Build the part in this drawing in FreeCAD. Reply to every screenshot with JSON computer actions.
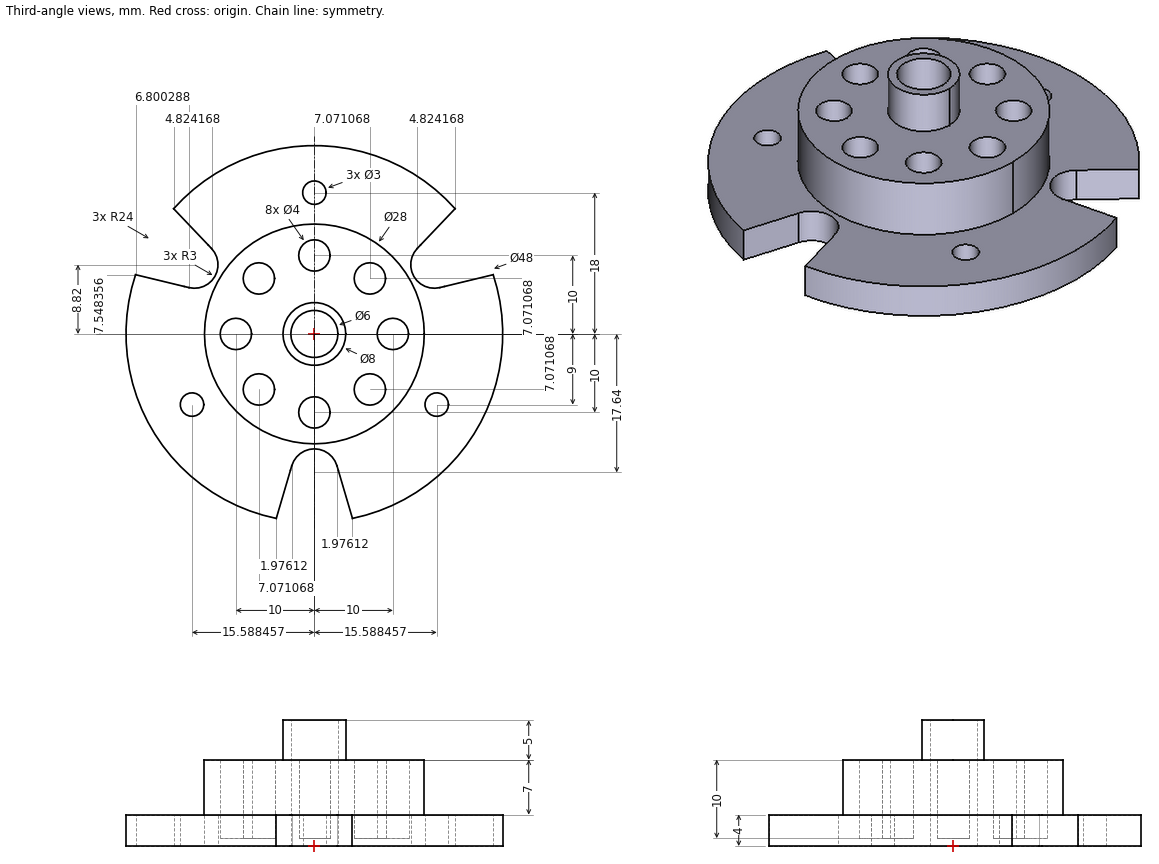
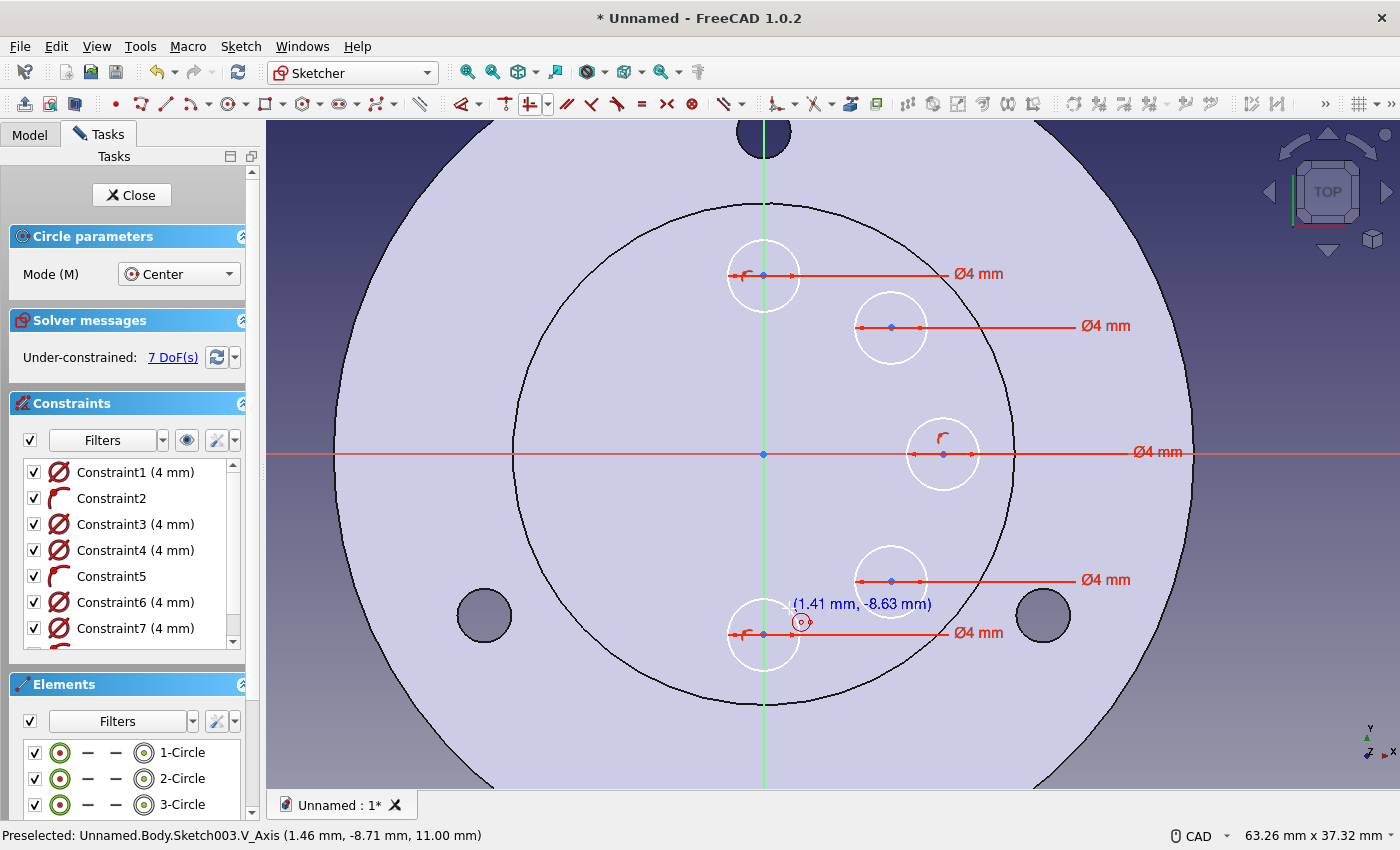
{"action": "left_click", "coordinate": [637, 581]}
{"action": "mouse_move", "coordinate": [662, 556]}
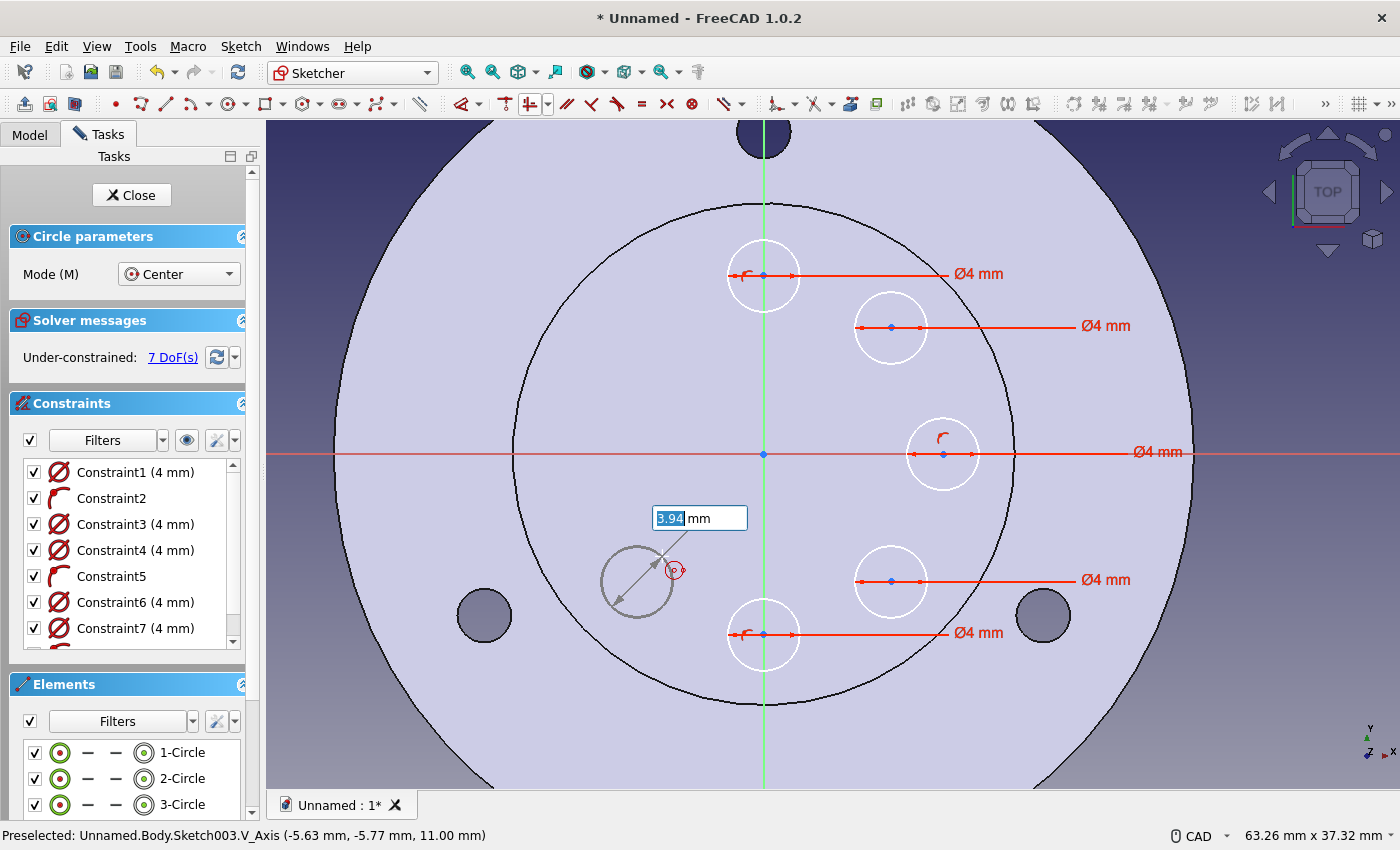
{"action": "type", "text": "4"}
{"action": "key", "text": "Return"}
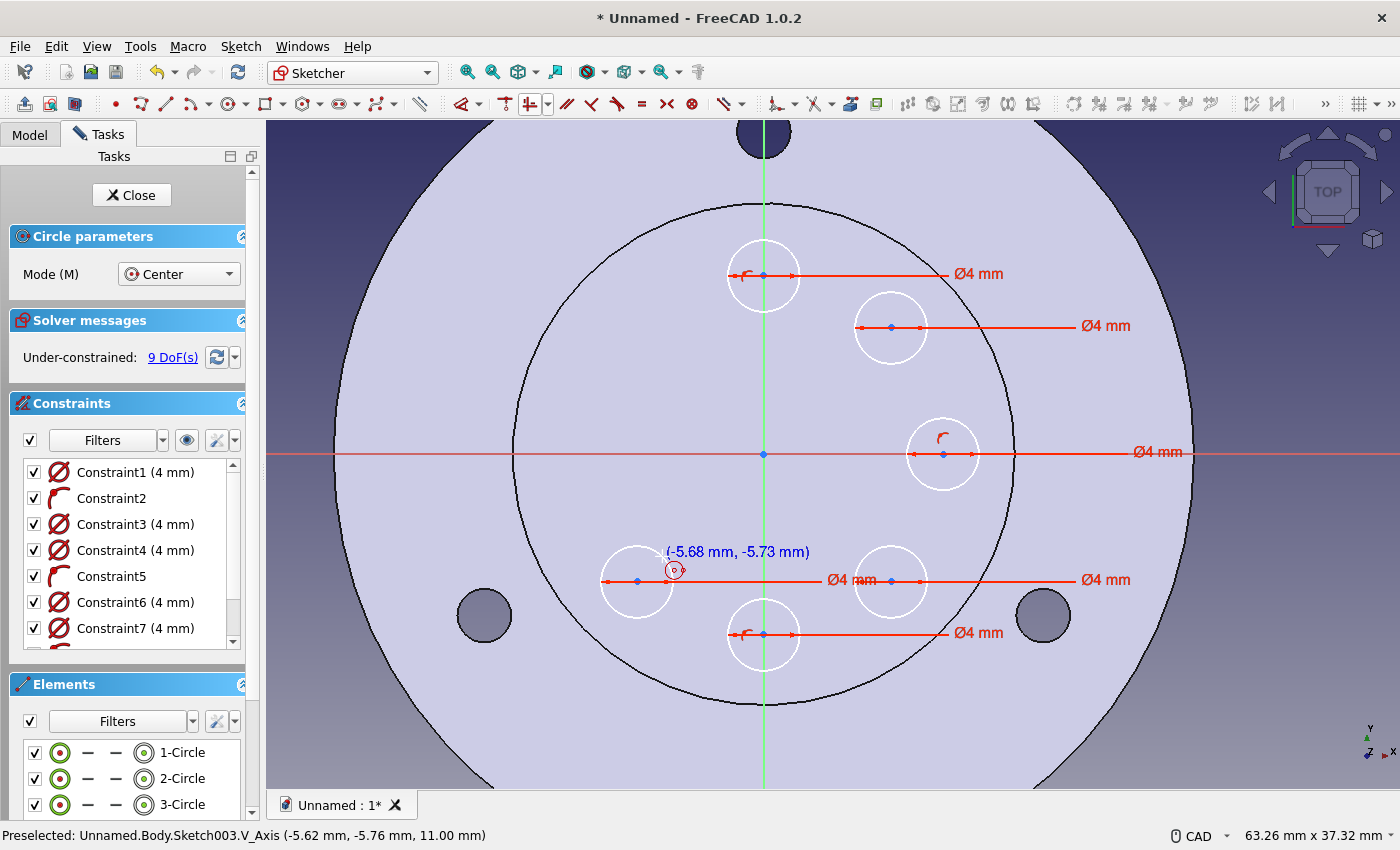
{"action": "left_click", "coordinate": [585, 454]}
{"action": "mouse_move", "coordinate": [610, 429]}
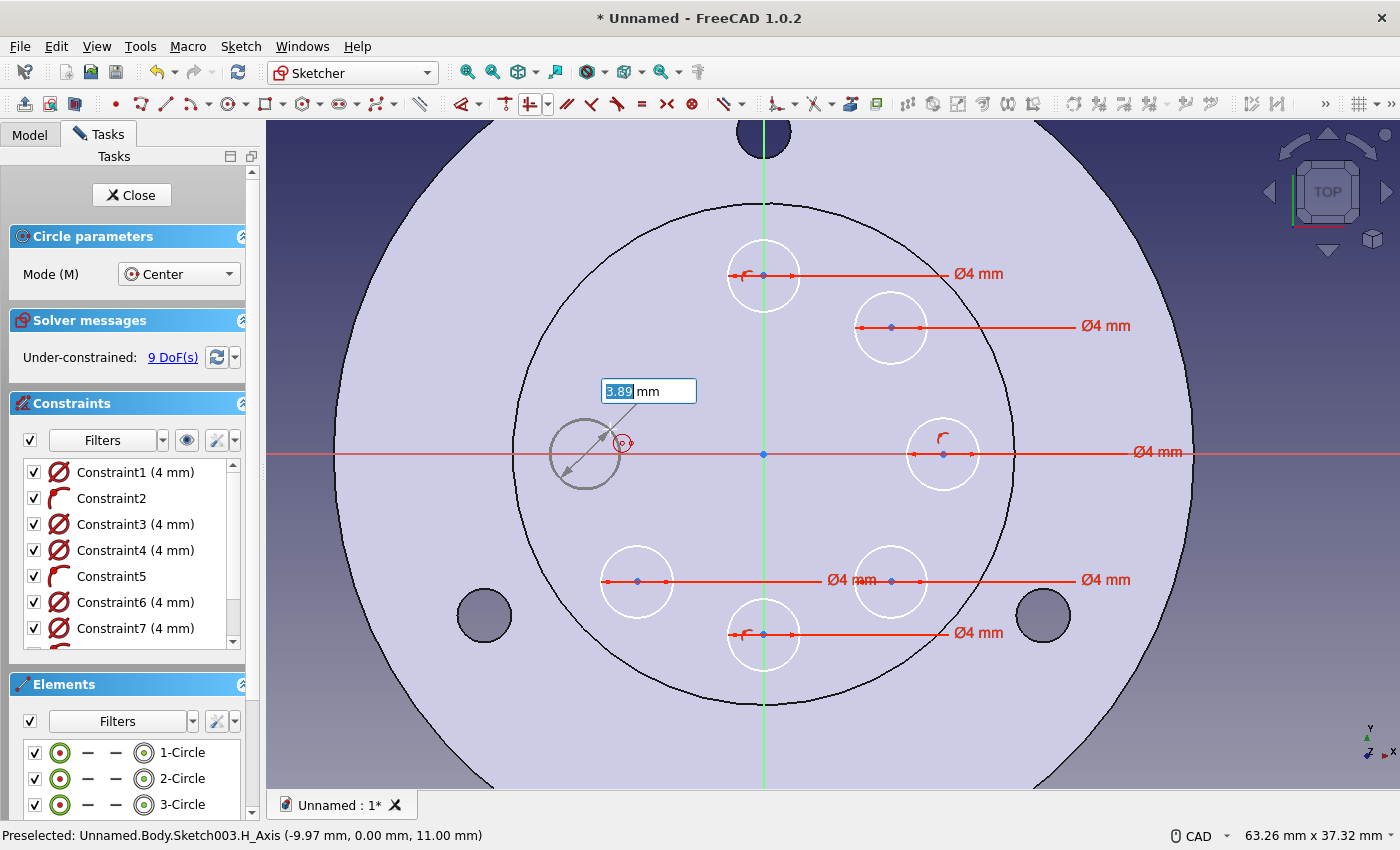
{"action": "type", "text": "4"}
{"action": "key", "text": "Return"}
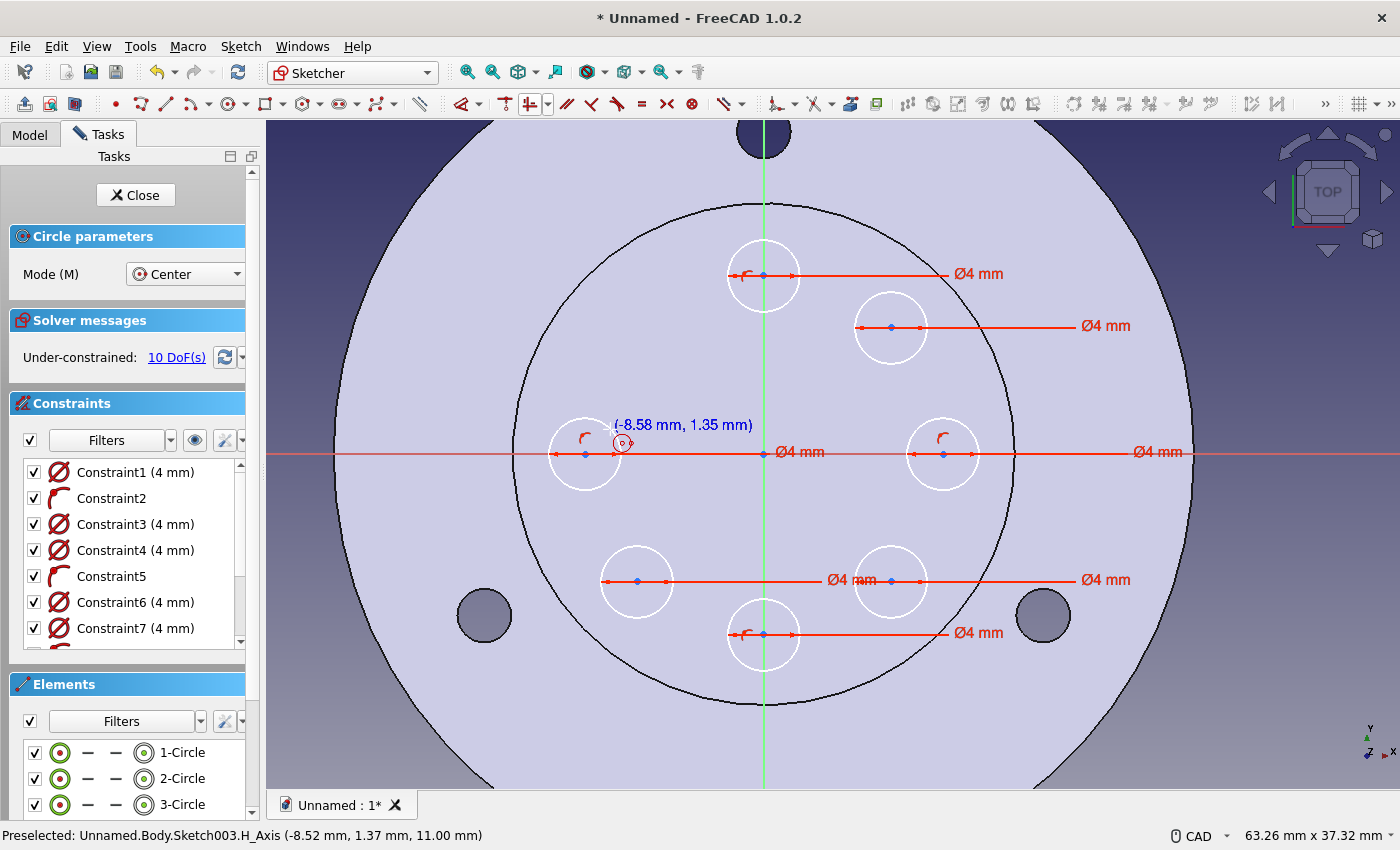
{"action": "left_click", "coordinate": [637, 327]}
{"action": "mouse_move", "coordinate": [662, 302]}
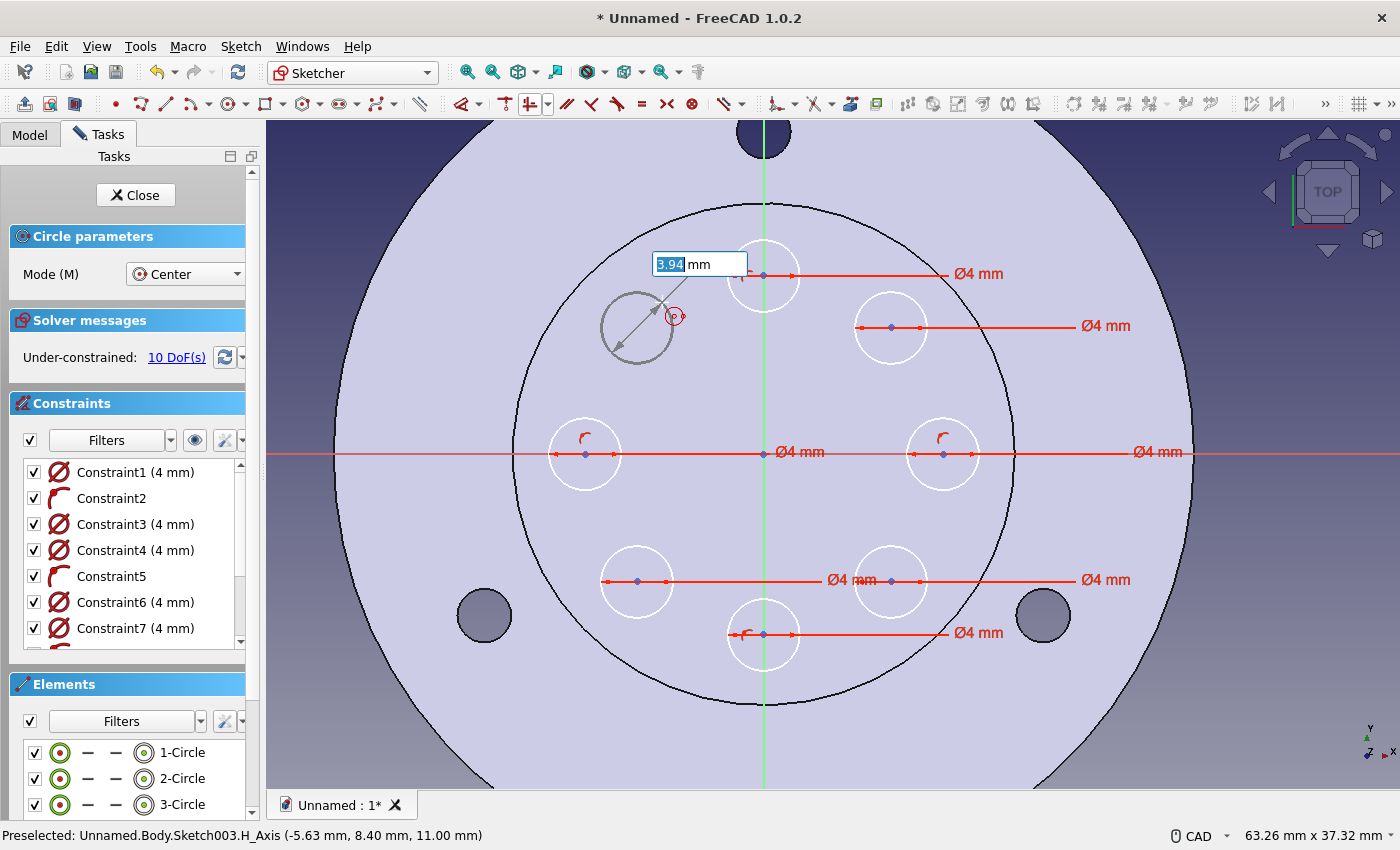
{"action": "type", "text": "4"}
{"action": "key", "text": "Return"}
{"action": "key", "text": "Escape"}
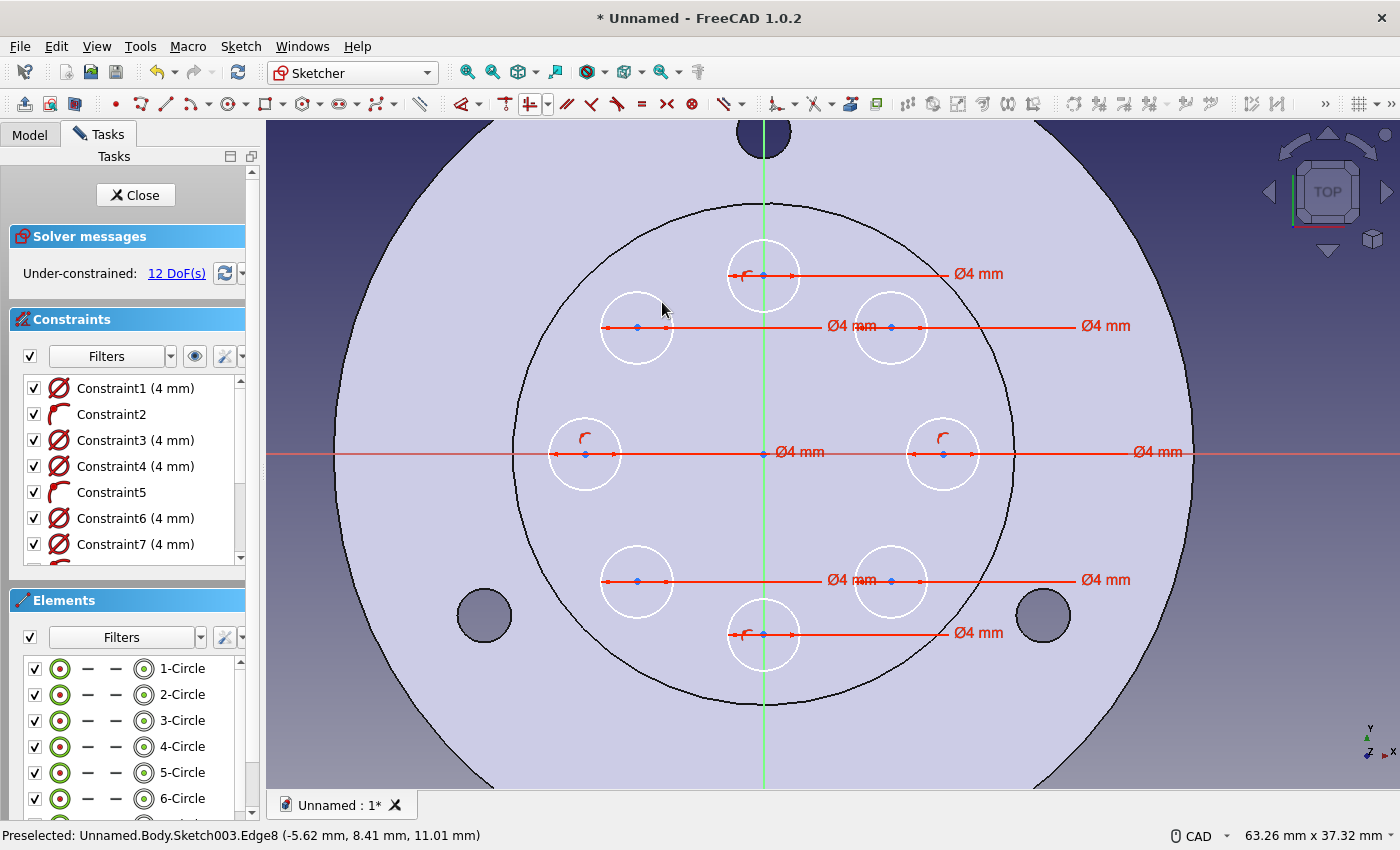
{"action": "left_click", "coordinate": [891, 328]}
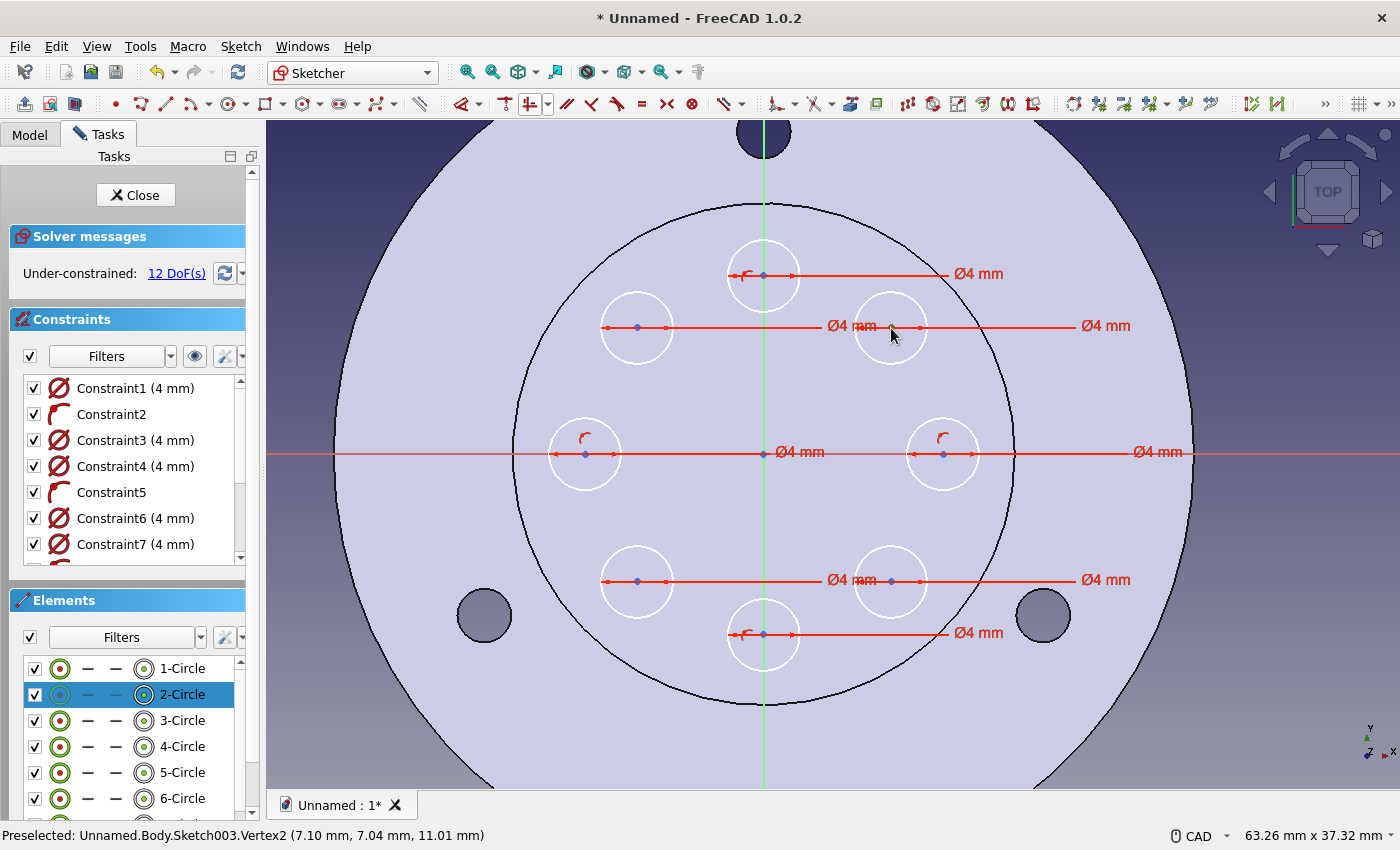
{"action": "left_click", "coordinate": [891, 582]}